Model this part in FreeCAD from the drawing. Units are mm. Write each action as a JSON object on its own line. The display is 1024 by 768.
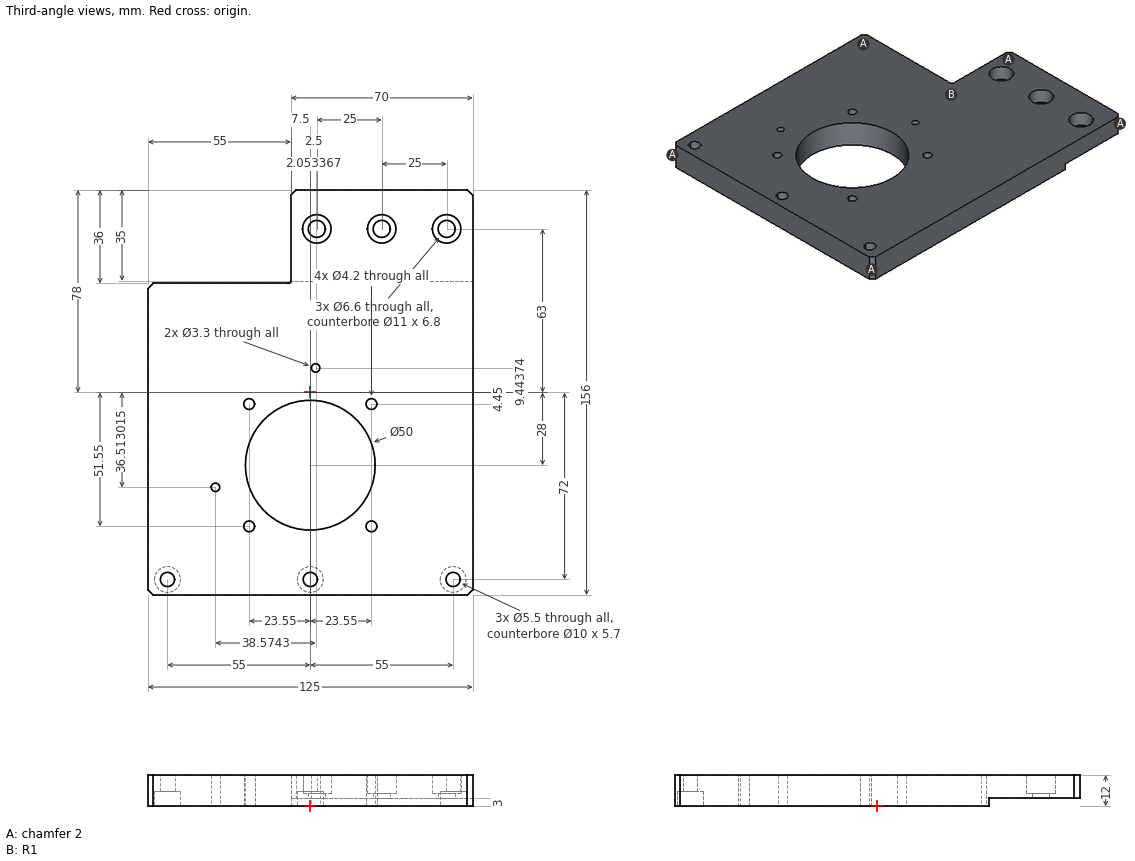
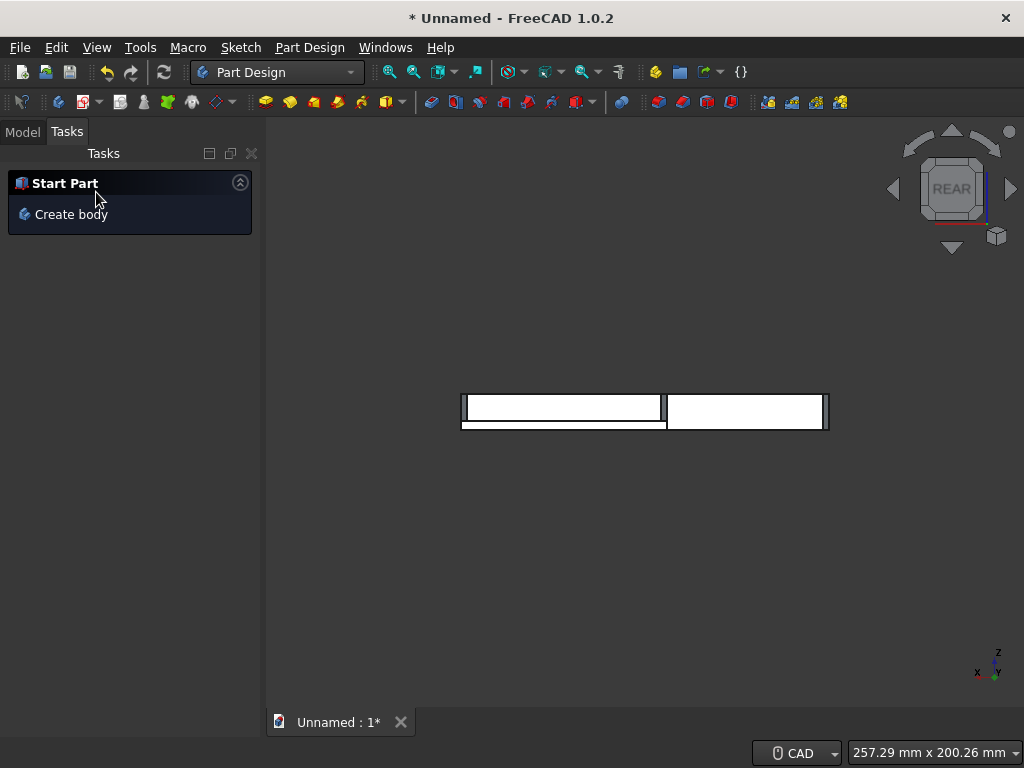
{"action": "key", "text": "6"}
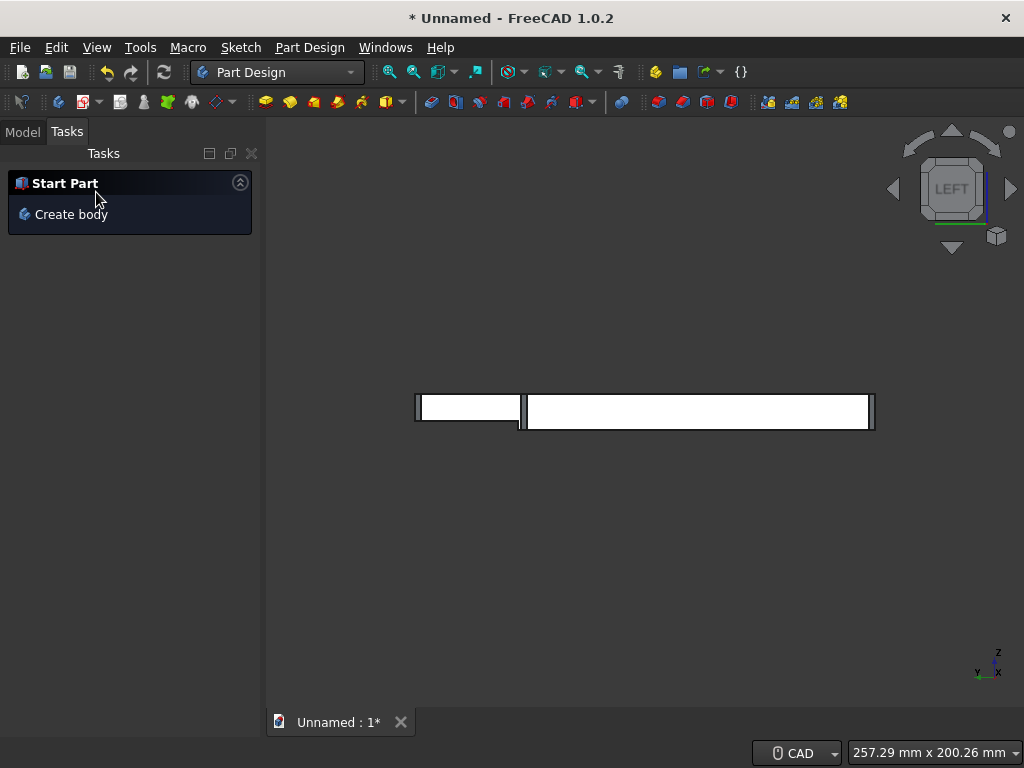
{"action": "key", "text": "v 3"}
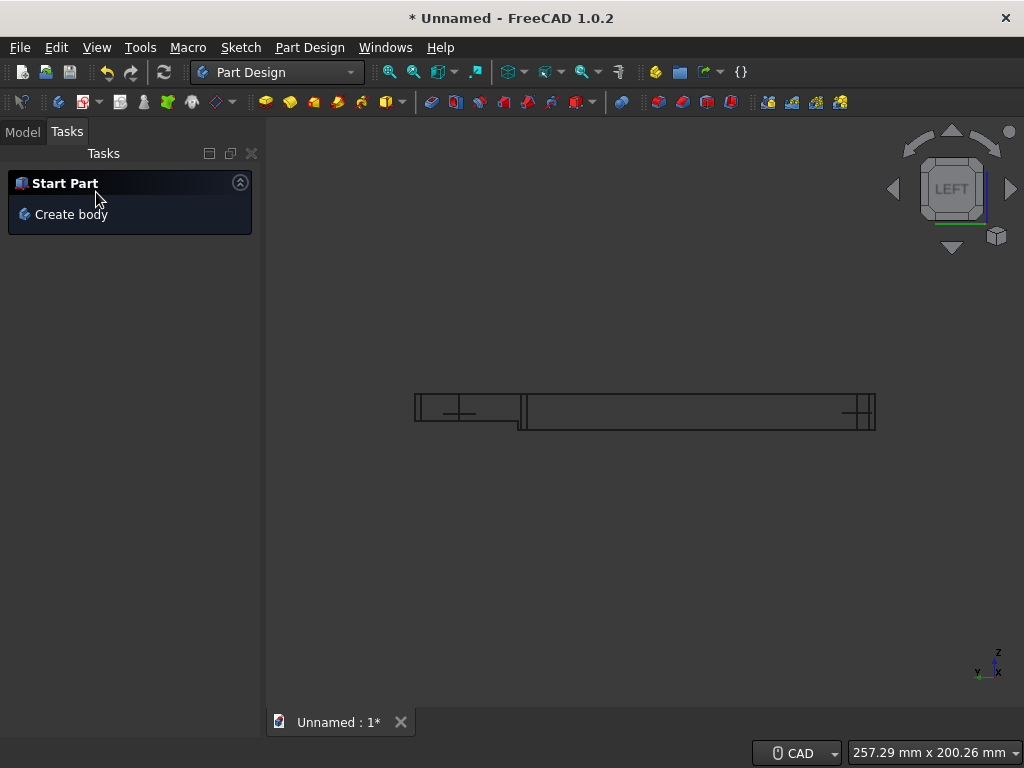
{"action": "key", "text": "0"}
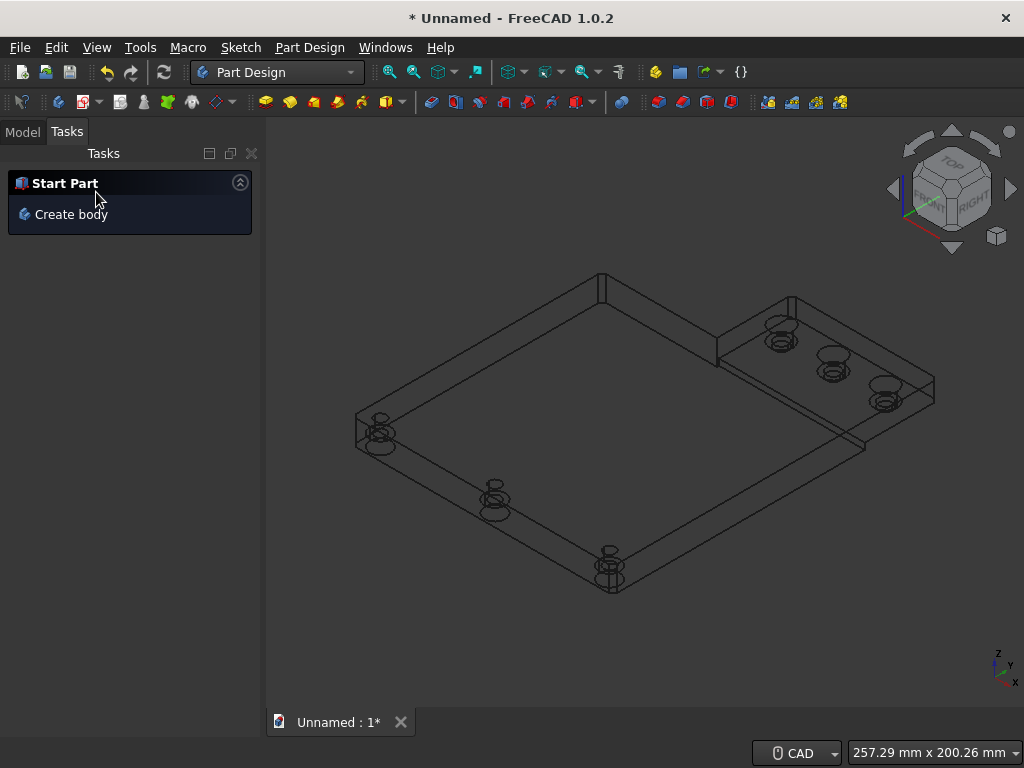
{"action": "left_click", "coordinate": [717, 351]}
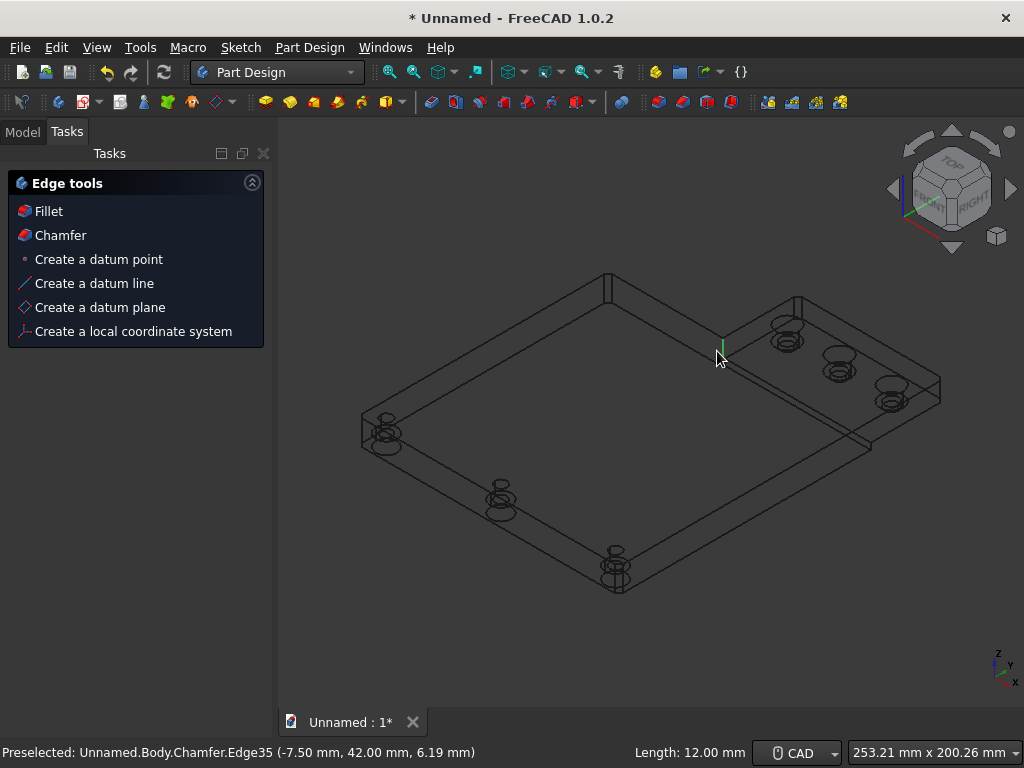
{"action": "key", "text": "v 1"}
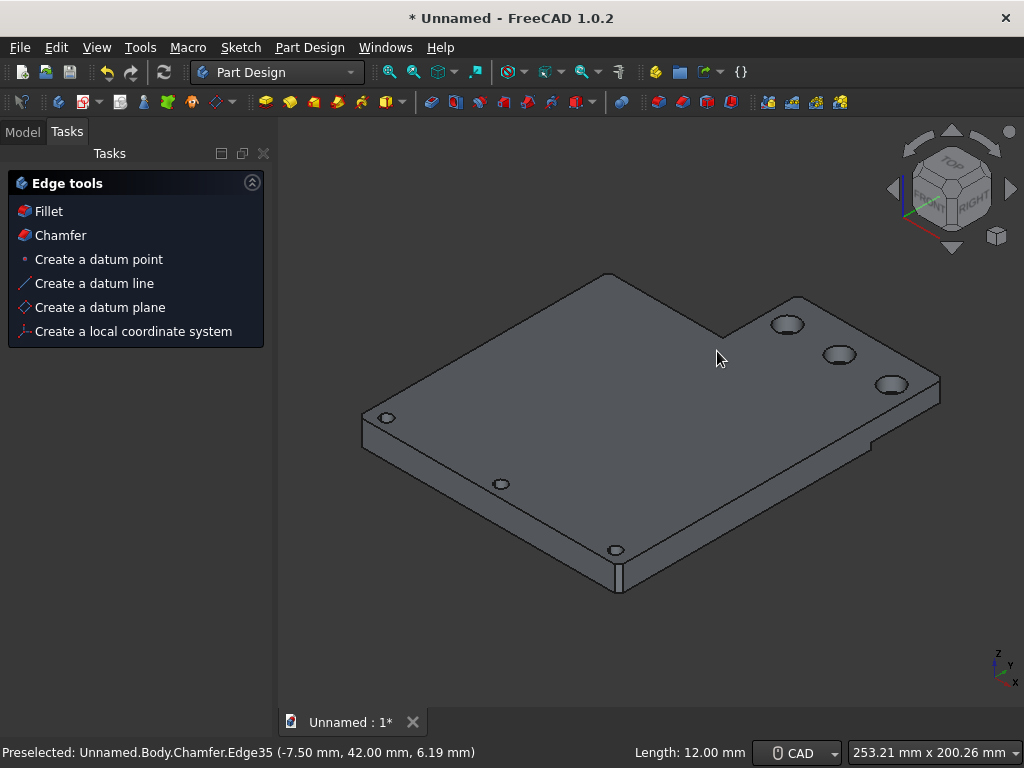
{"action": "left_click", "coordinate": [660, 102]}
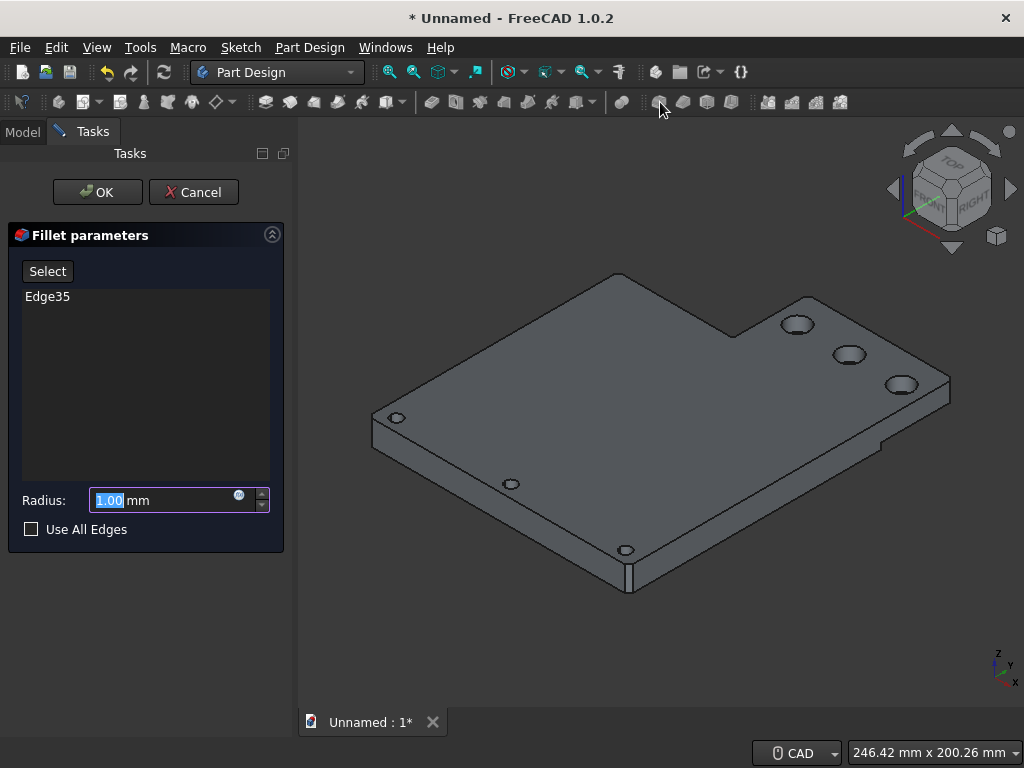
{"action": "type", "text": "1"}
{"action": "key", "text": "Tab"}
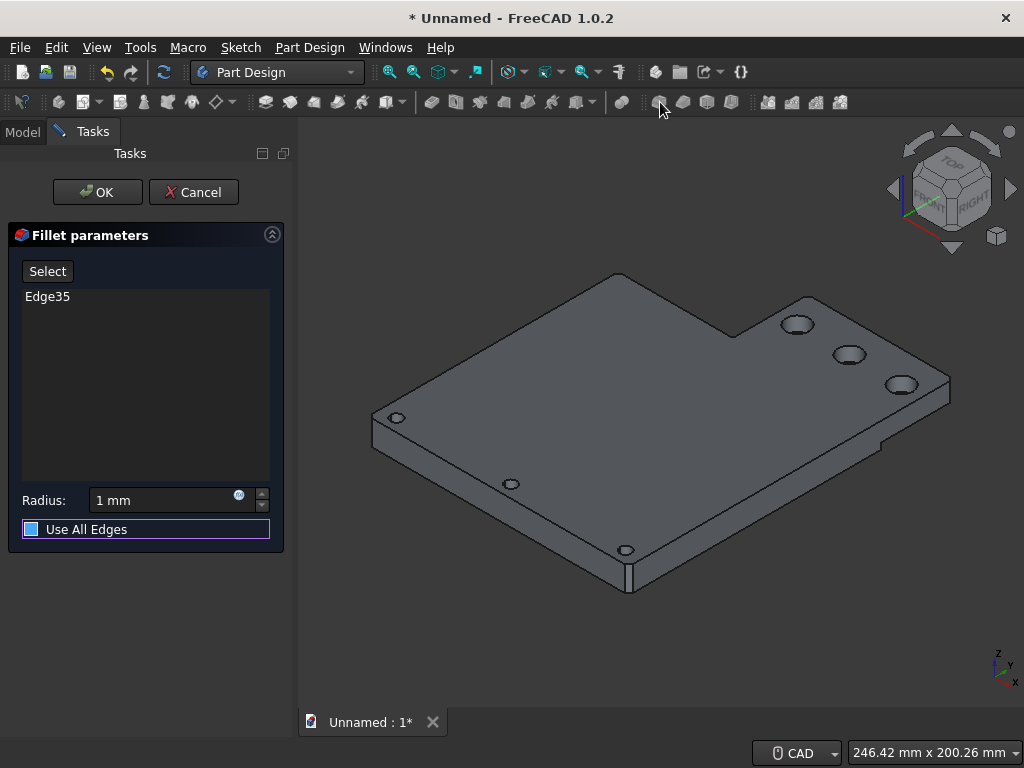
{"action": "left_click", "coordinate": [98, 192]}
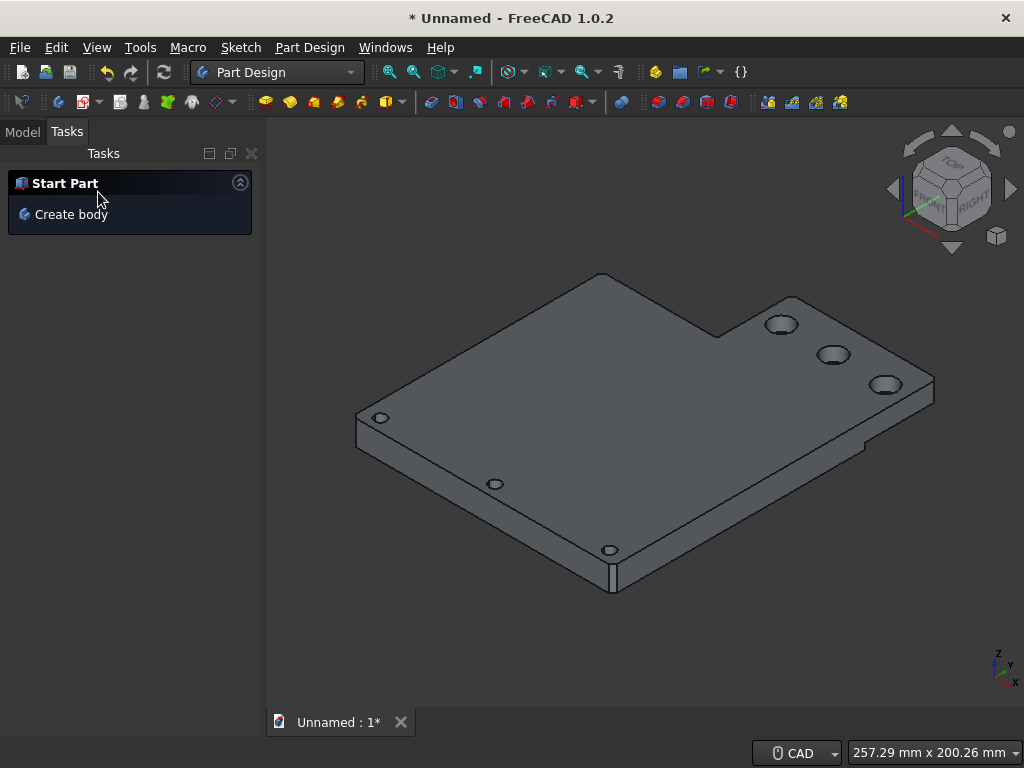
{"action": "left_click", "coordinate": [599, 423]}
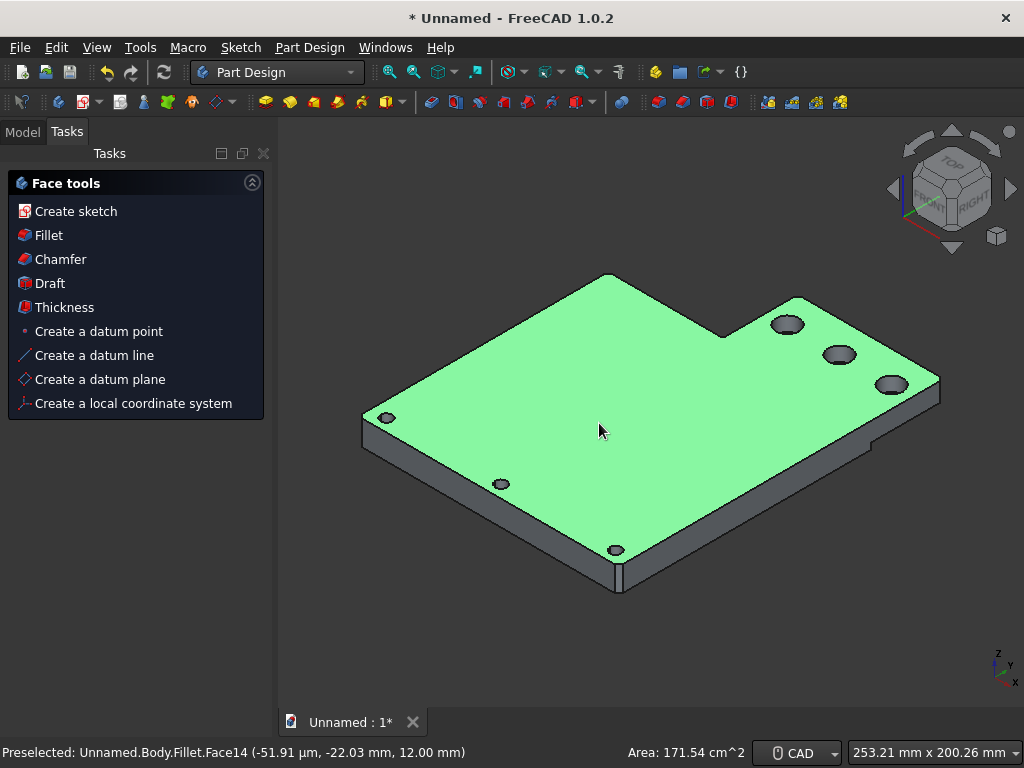
{"action": "left_click", "coordinate": [84, 102]}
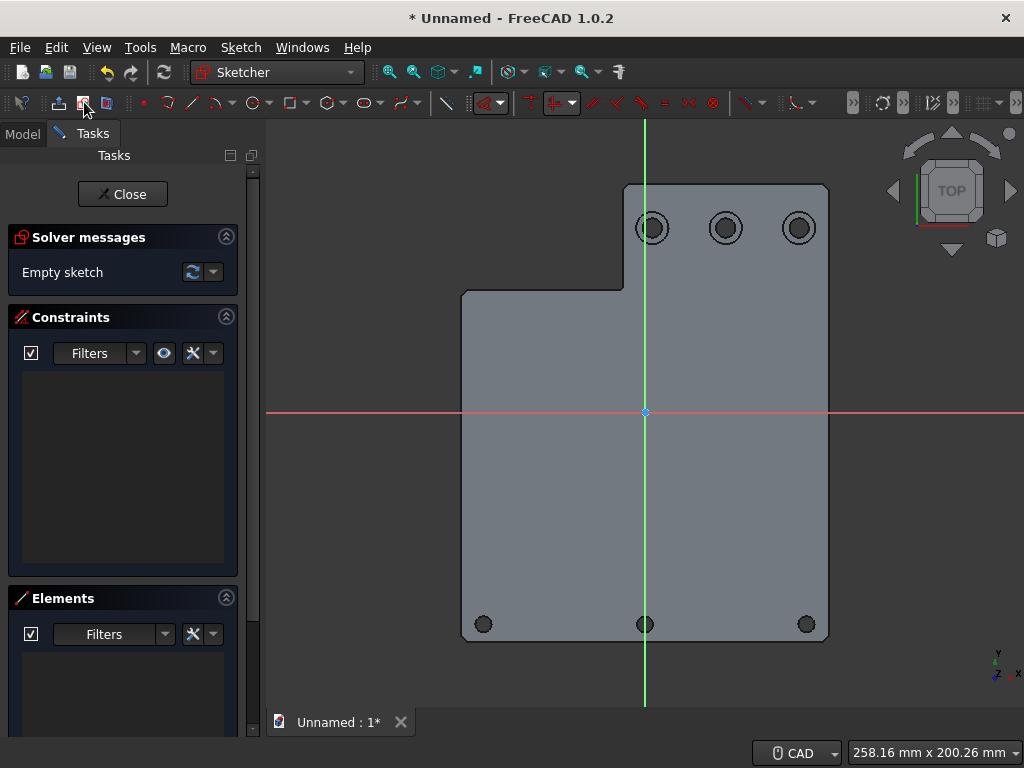
{"action": "scroll", "coordinate": [701, 554], "scroll_direction": "up", "scroll_amount": 4}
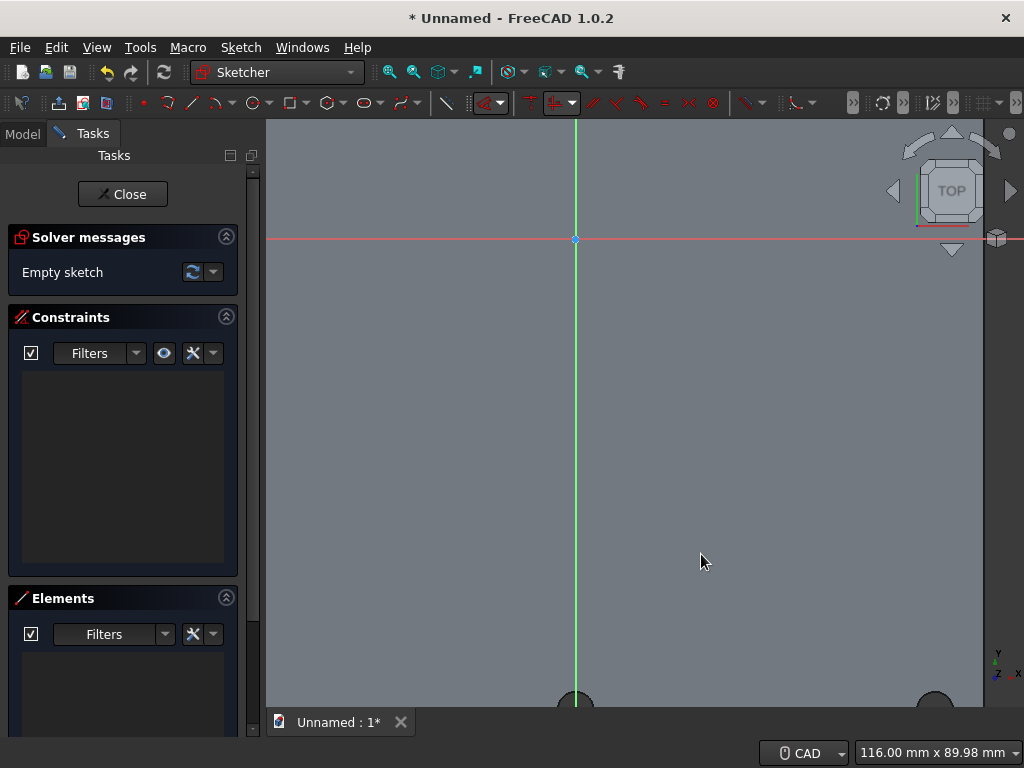
{"action": "left_click", "coordinate": [254, 104]}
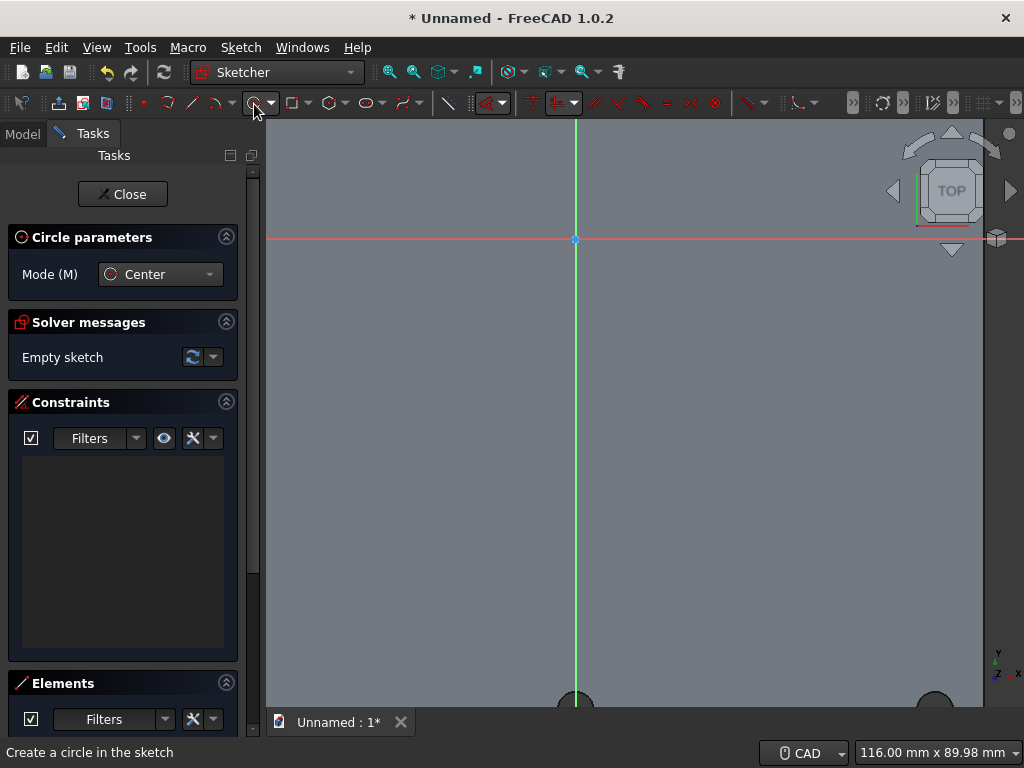
{"action": "left_click", "coordinate": [576, 422]}
{"action": "left_click", "coordinate": [691, 307]}
{"action": "key", "text": "Escape"}